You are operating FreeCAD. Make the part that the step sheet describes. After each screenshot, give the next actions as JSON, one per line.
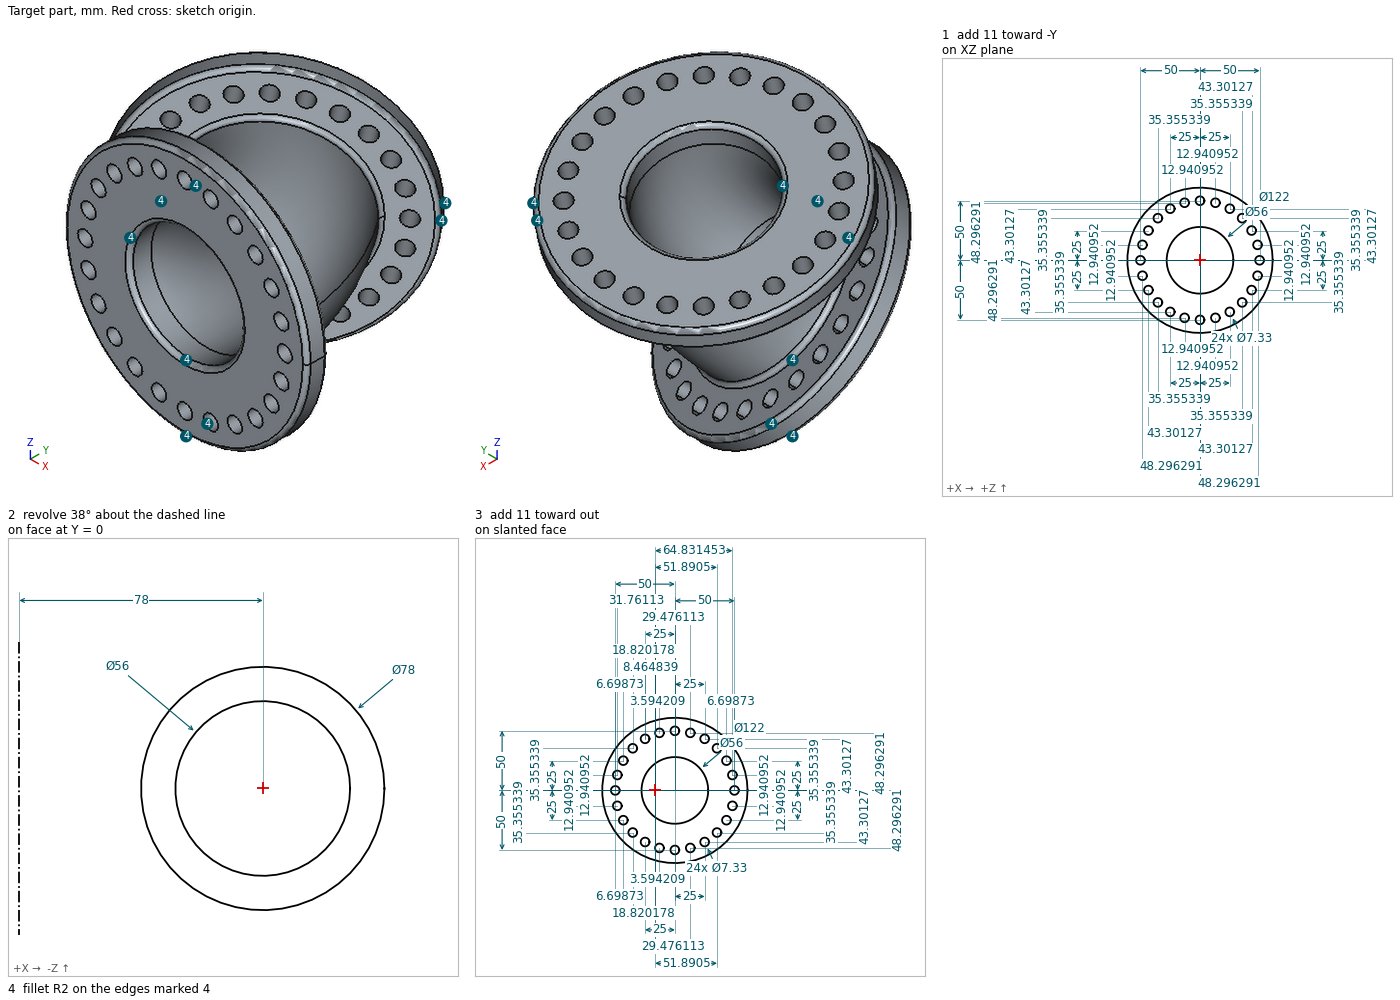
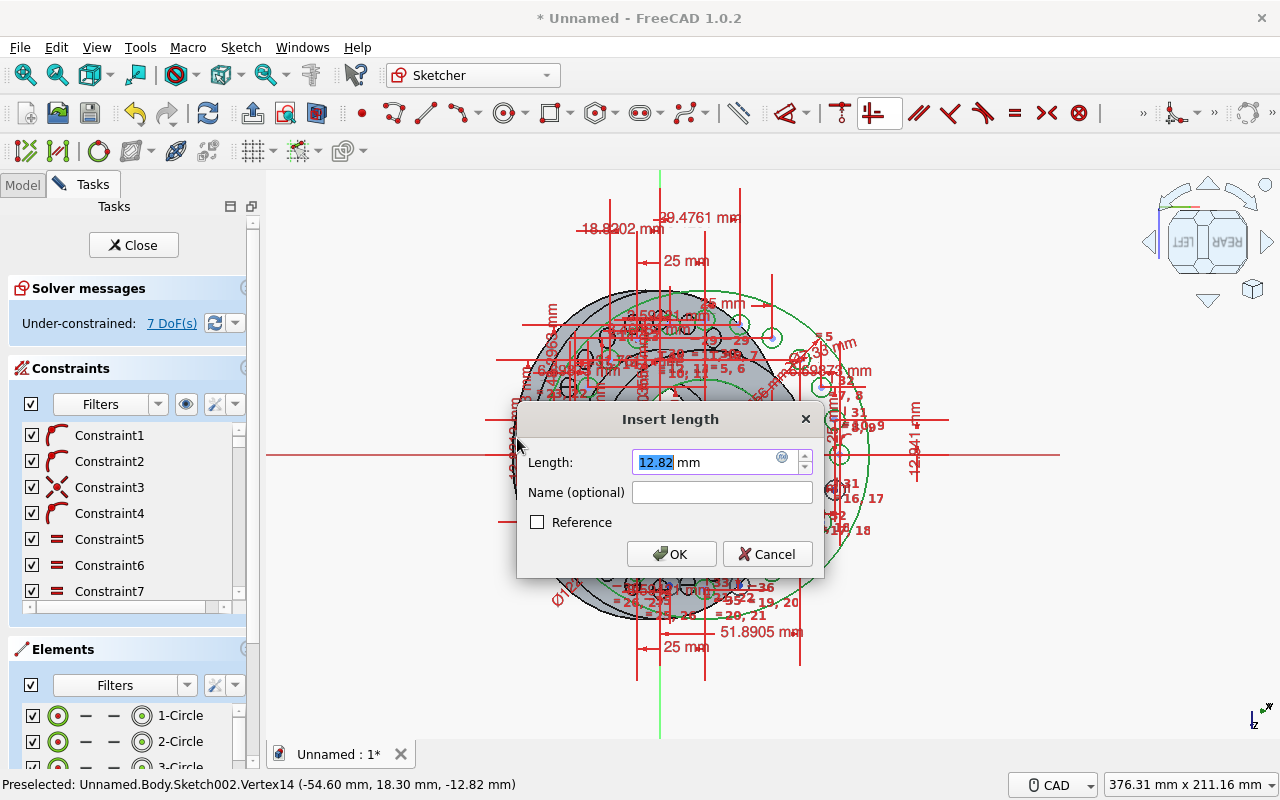
{"action": "type", "text": "12.940952"}
{"action": "key", "text": "Return"}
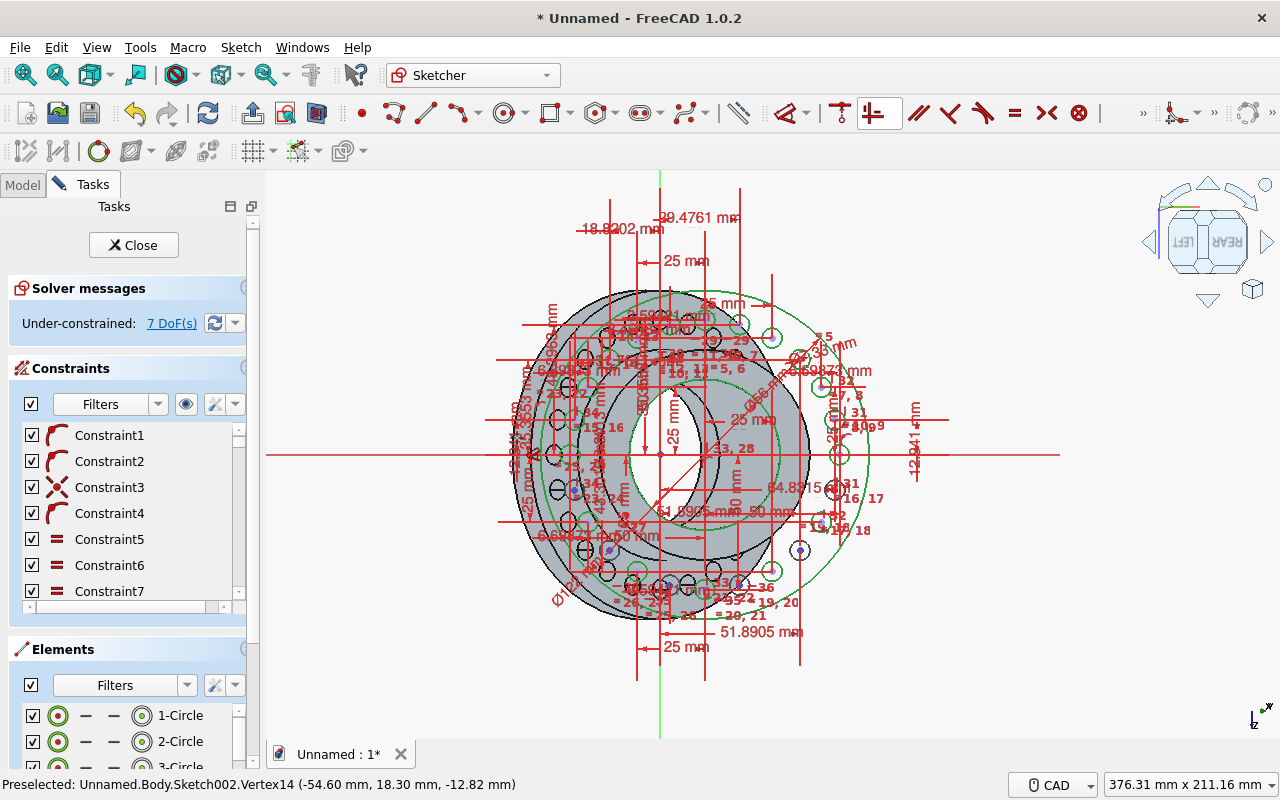
{"action": "left_click", "coordinate": [835, 490]}
{"action": "left_click", "coordinate": [893, 472]}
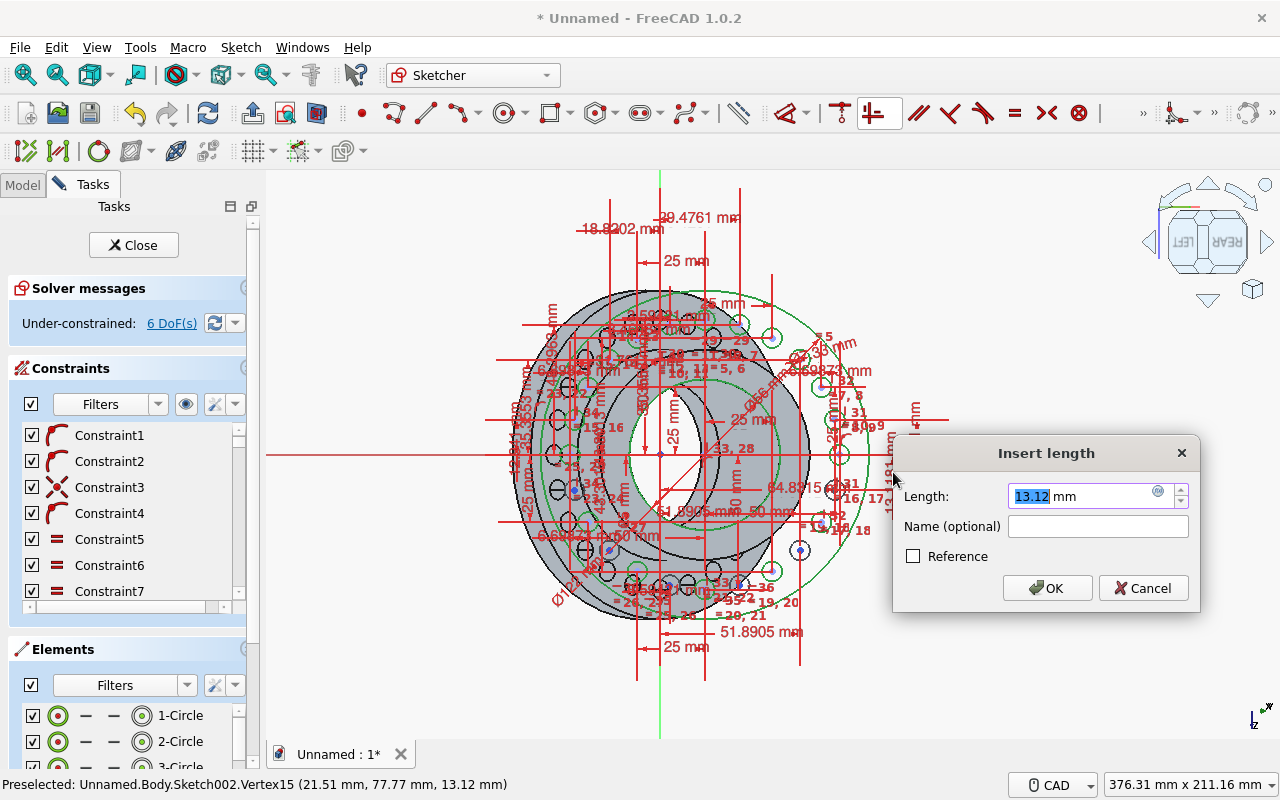
{"action": "type", "text": "12.940952"}
{"action": "key", "text": "Return"}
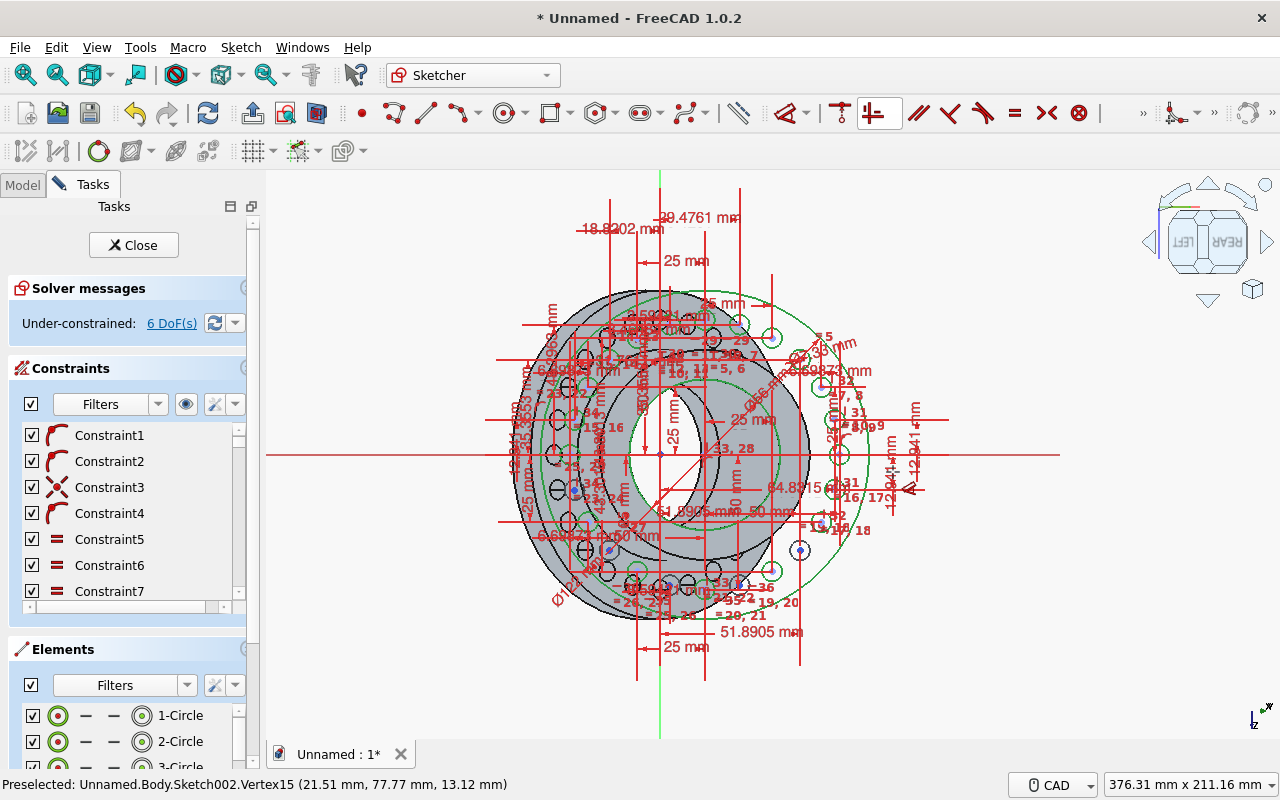
{"action": "left_click", "coordinate": [800, 551]}
{"action": "left_click", "coordinate": [882, 503]}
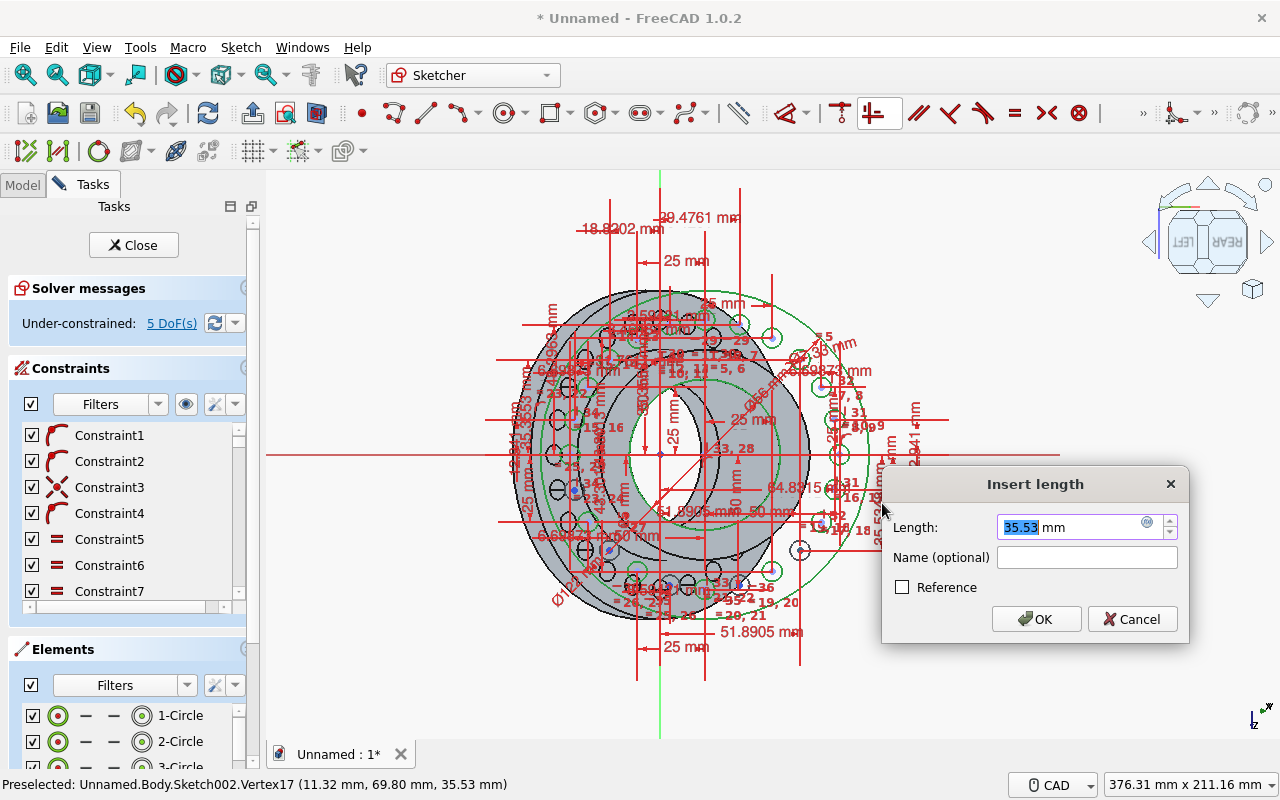
{"action": "type", "text": "35.355339"}
{"action": "key", "text": "Return"}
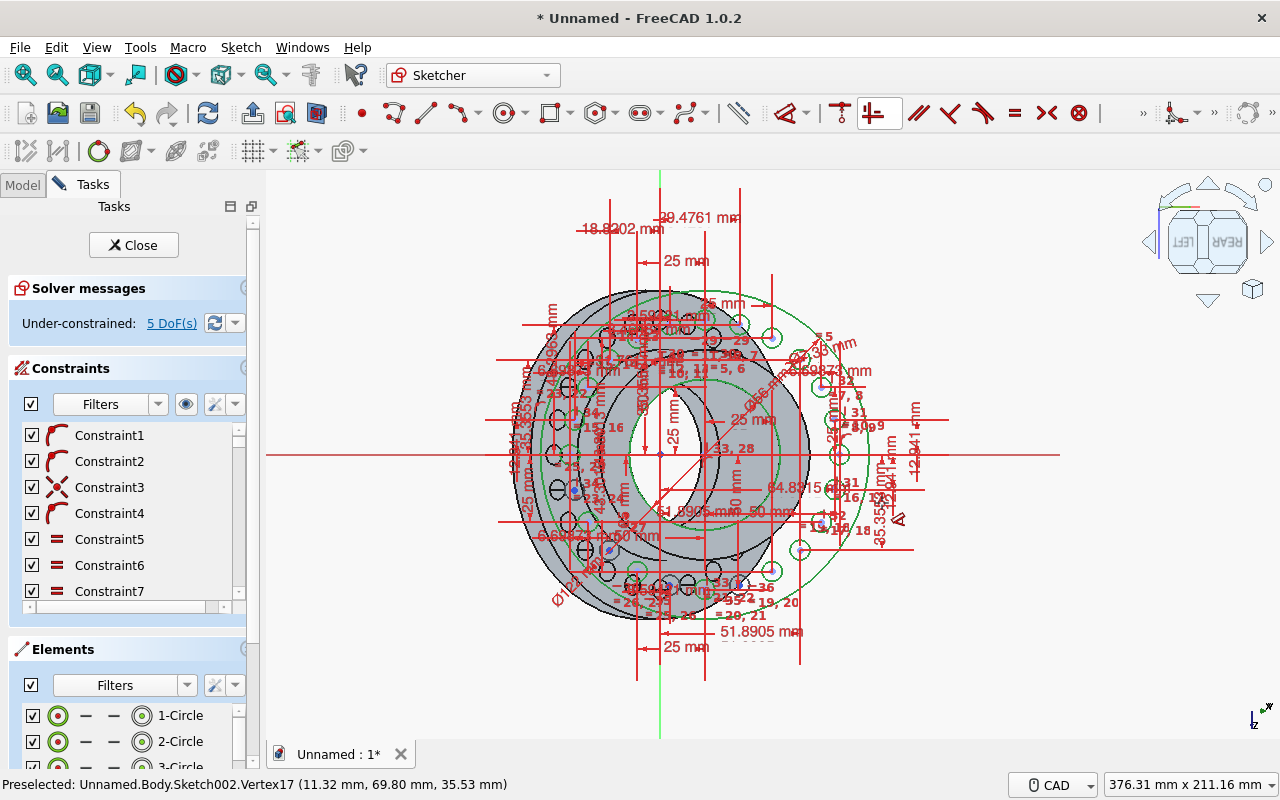
{"action": "left_click", "coordinate": [740, 585]}
{"action": "left_click", "coordinate": [700, 691]}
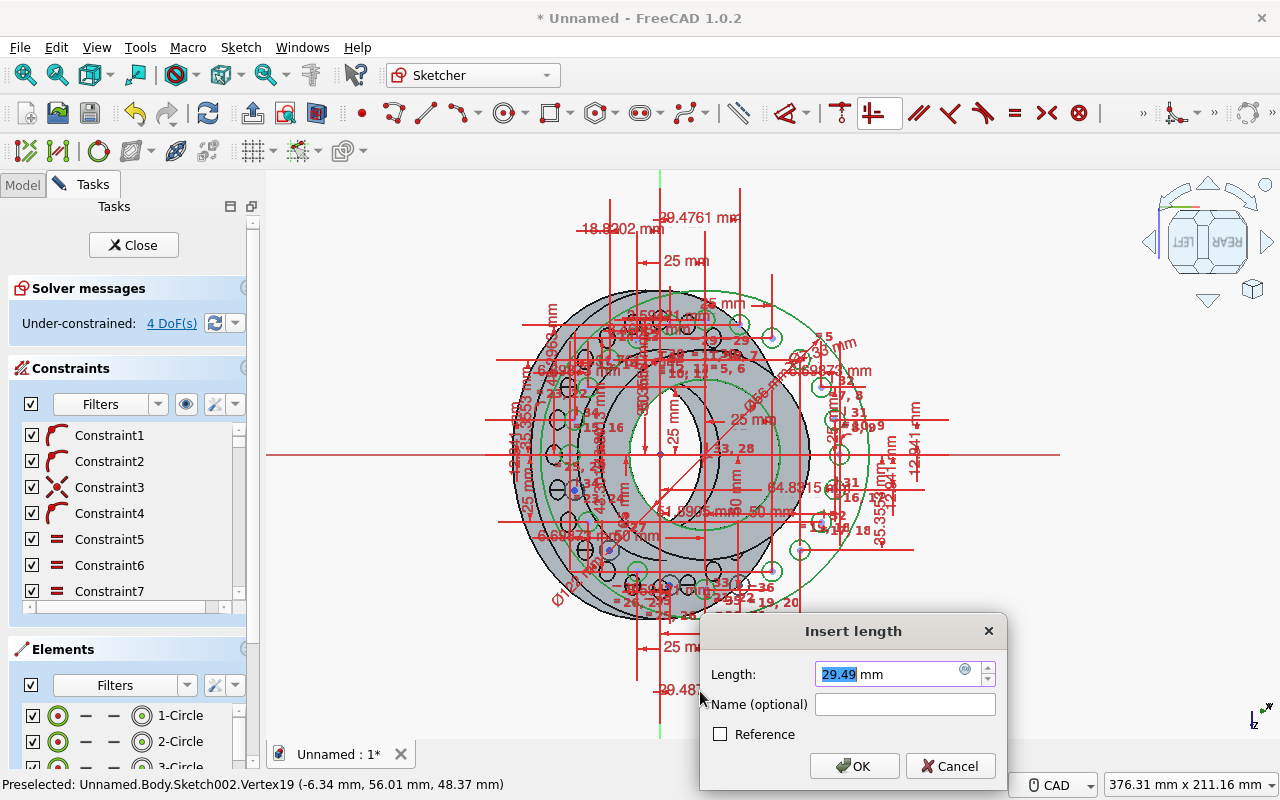
{"action": "type", "text": "29.476113"}
{"action": "key", "text": "Return"}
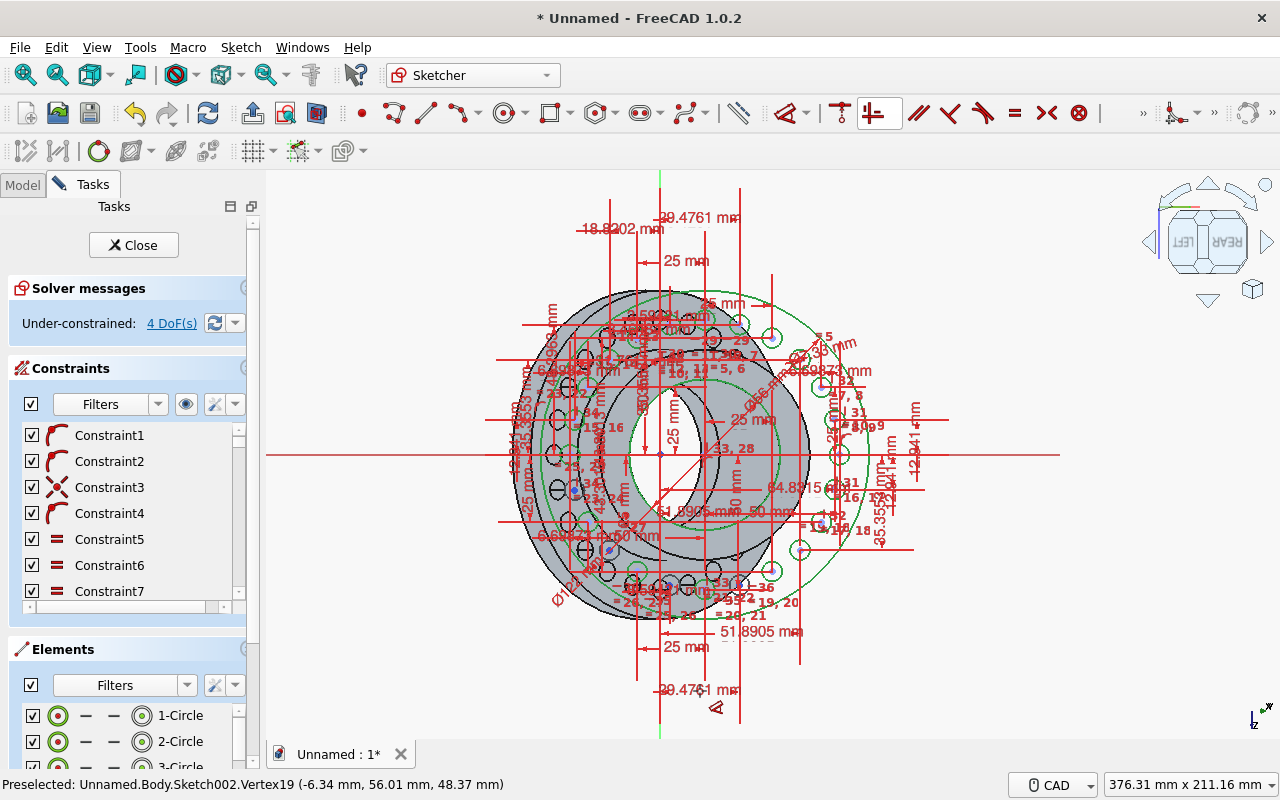
{"action": "left_click", "coordinate": [740, 585]}
{"action": "left_click", "coordinate": [846, 566]}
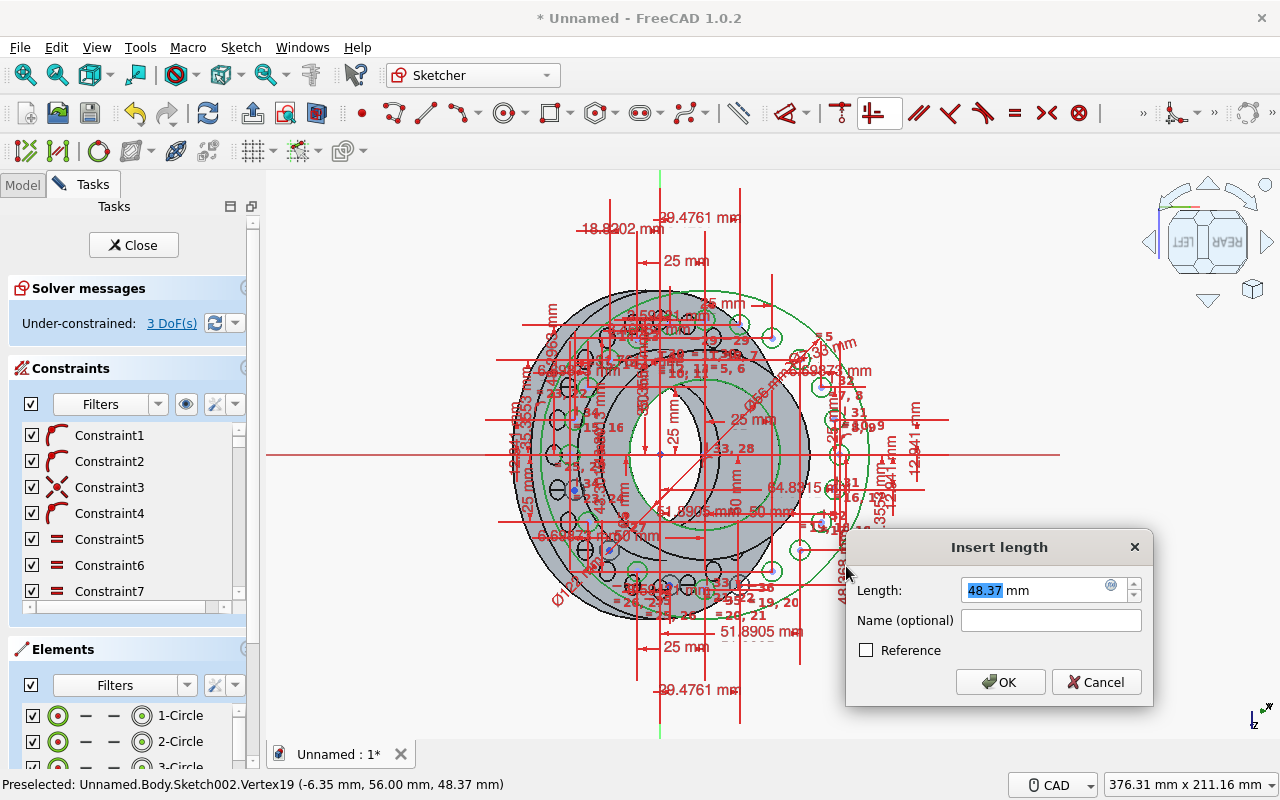
{"action": "type", "text": "48.296291"}
{"action": "key", "text": "Return"}